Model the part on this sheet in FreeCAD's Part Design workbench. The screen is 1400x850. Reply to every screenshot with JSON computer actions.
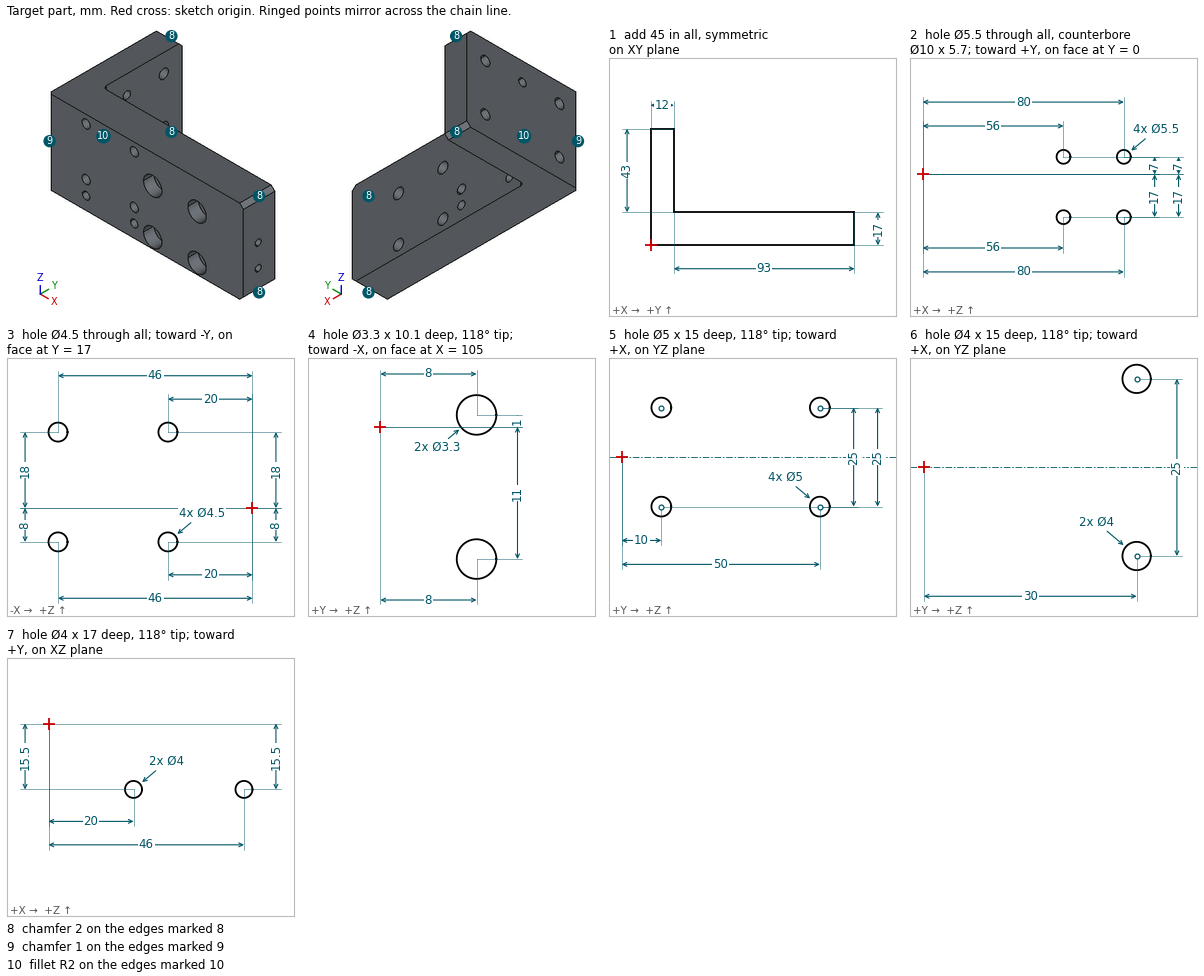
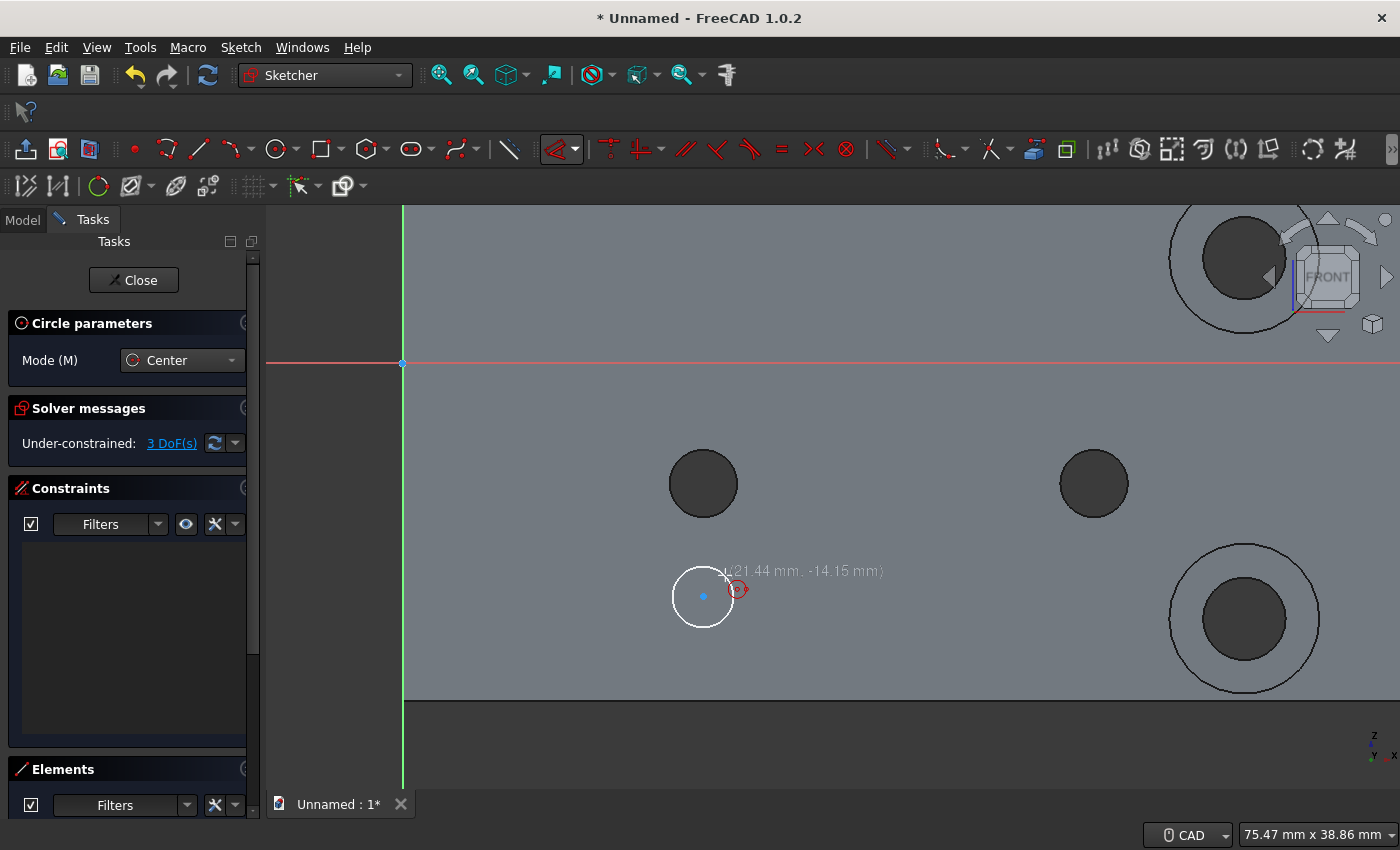
{"action": "left_click", "coordinate": [1094, 596]}
{"action": "left_click", "coordinate": [1115, 575]}
{"action": "key", "text": "Escape"}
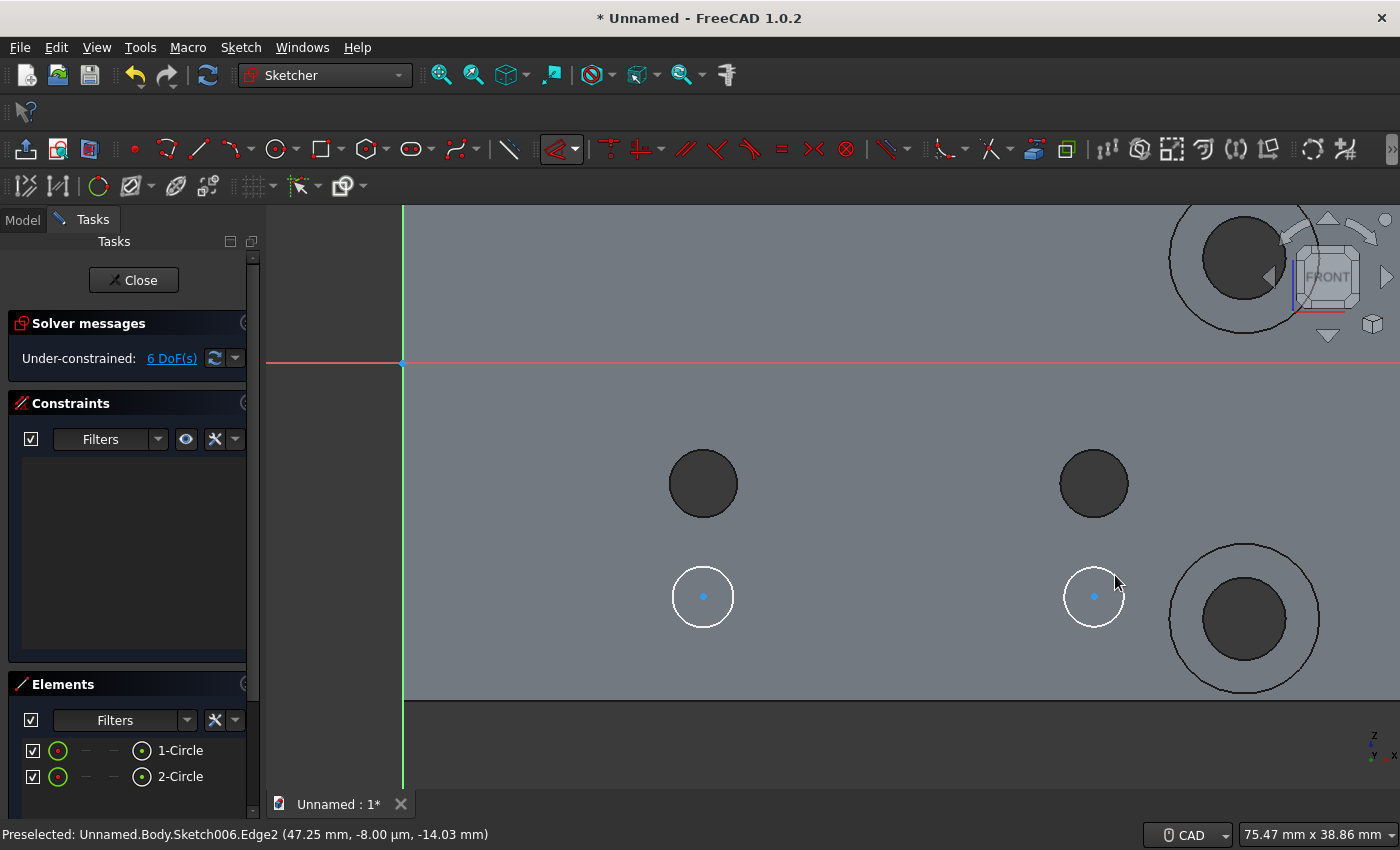
{"action": "left_click", "coordinate": [724, 575]}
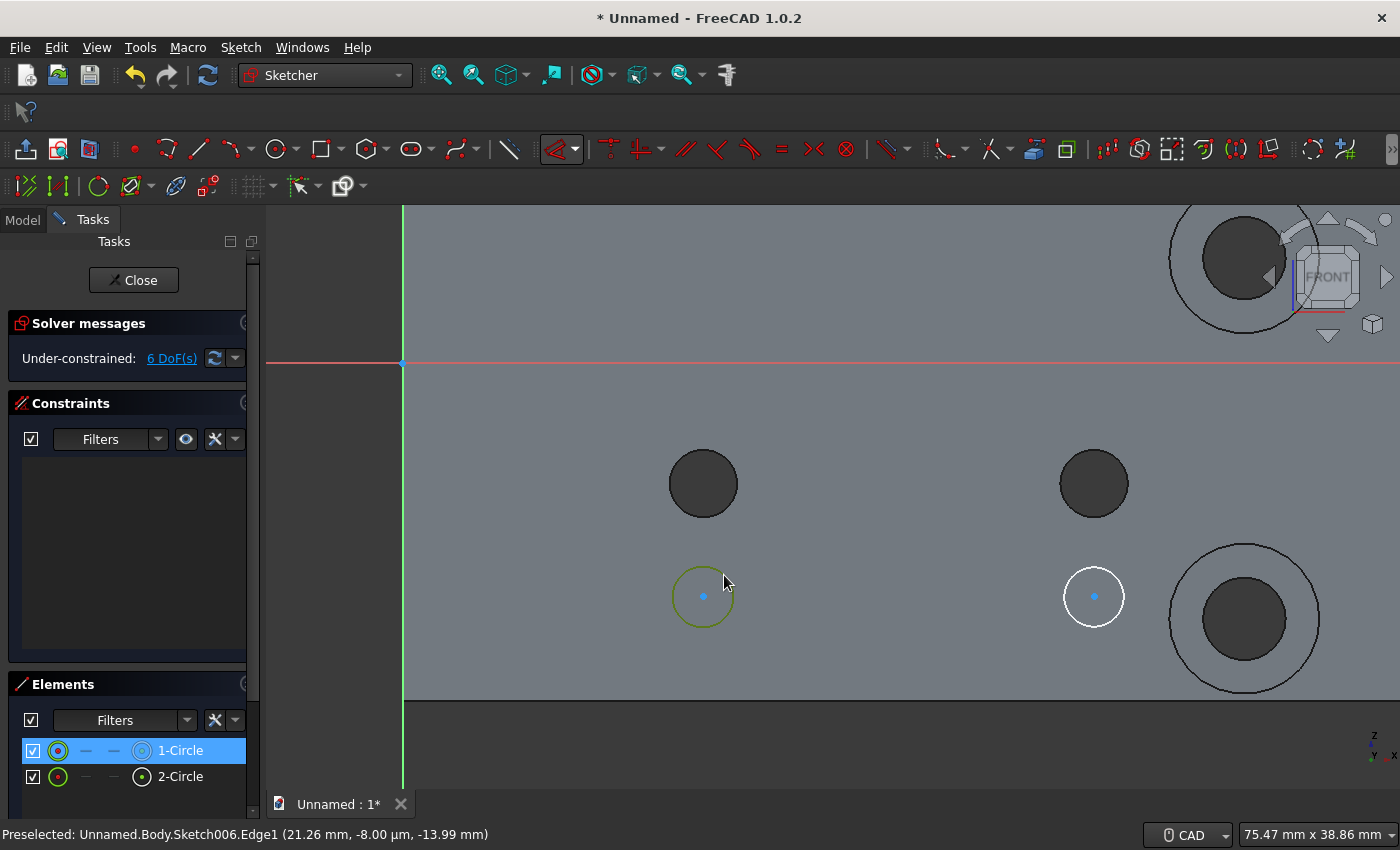
{"action": "left_click", "coordinate": [1115, 576]}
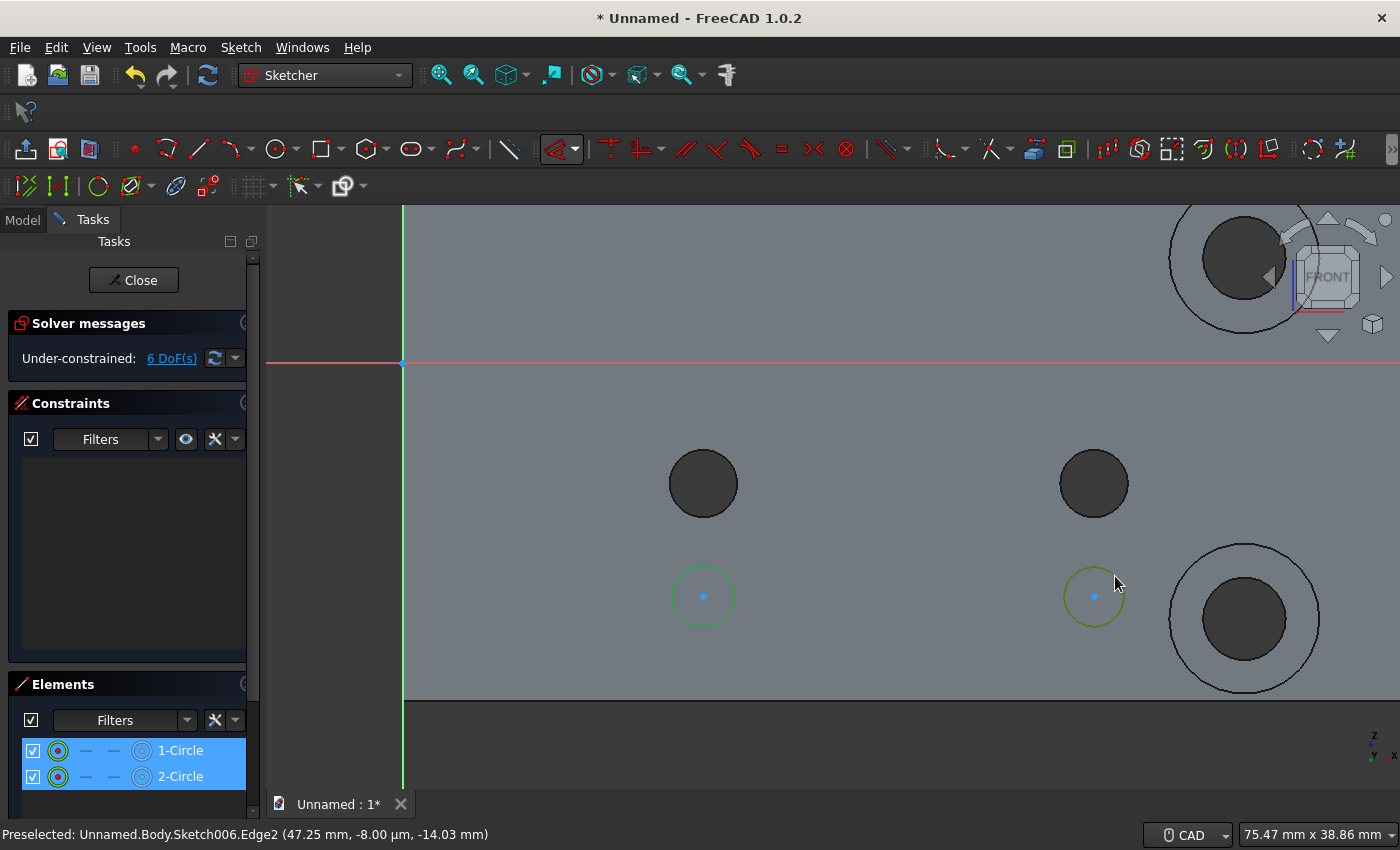
{"action": "key", "text": "e"}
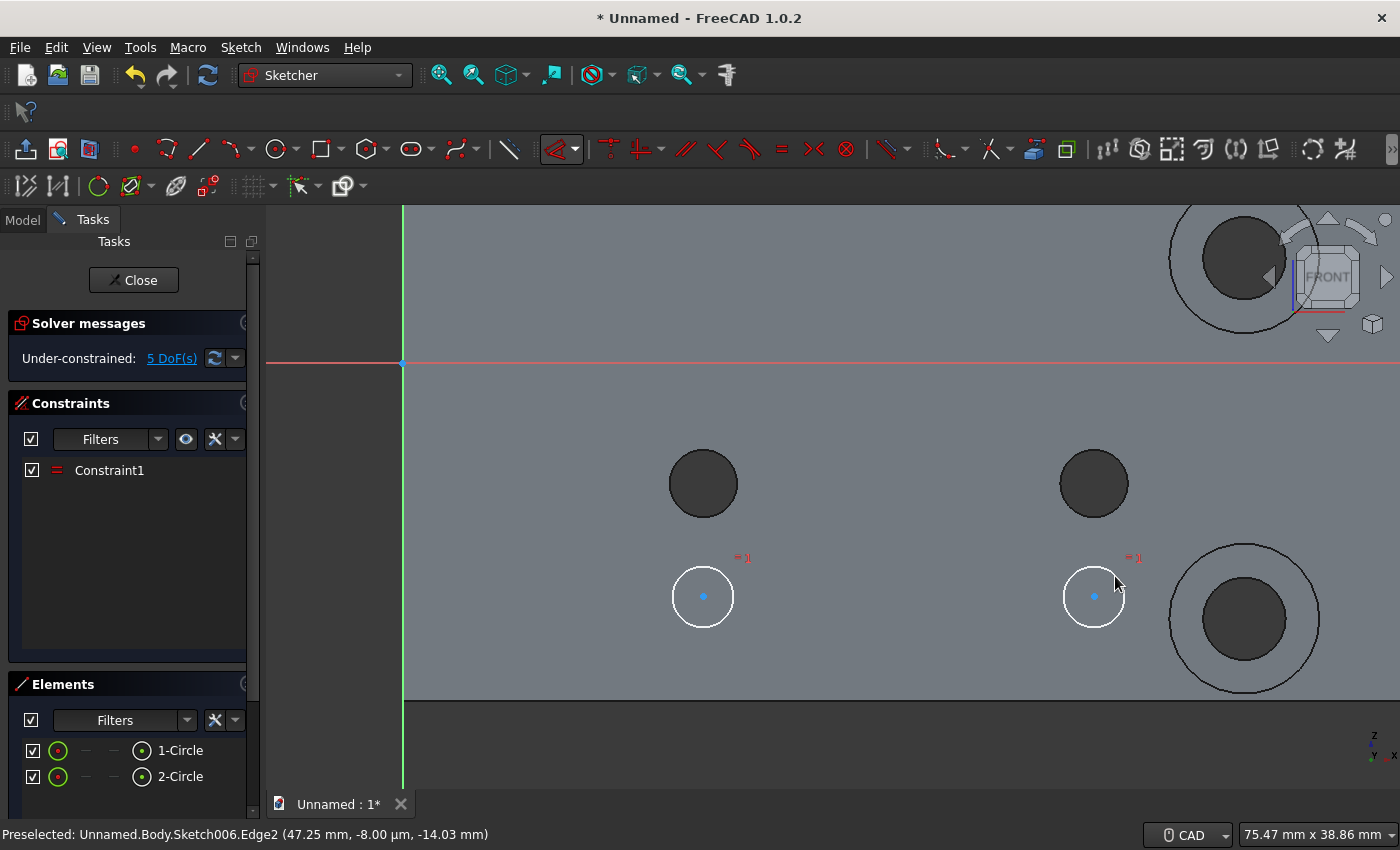
{"action": "left_click", "coordinate": [724, 575]}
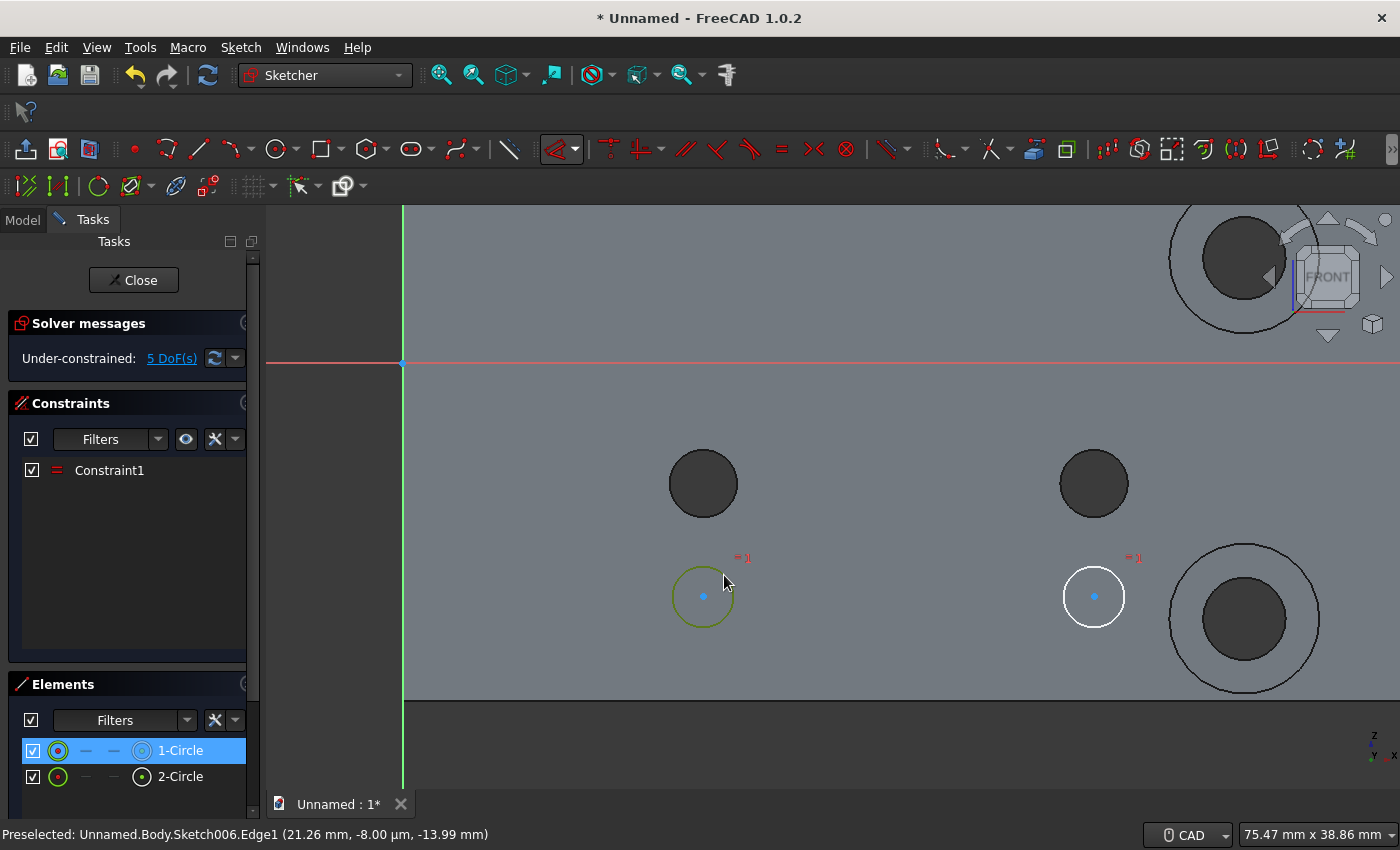
{"action": "key", "text": "k o"}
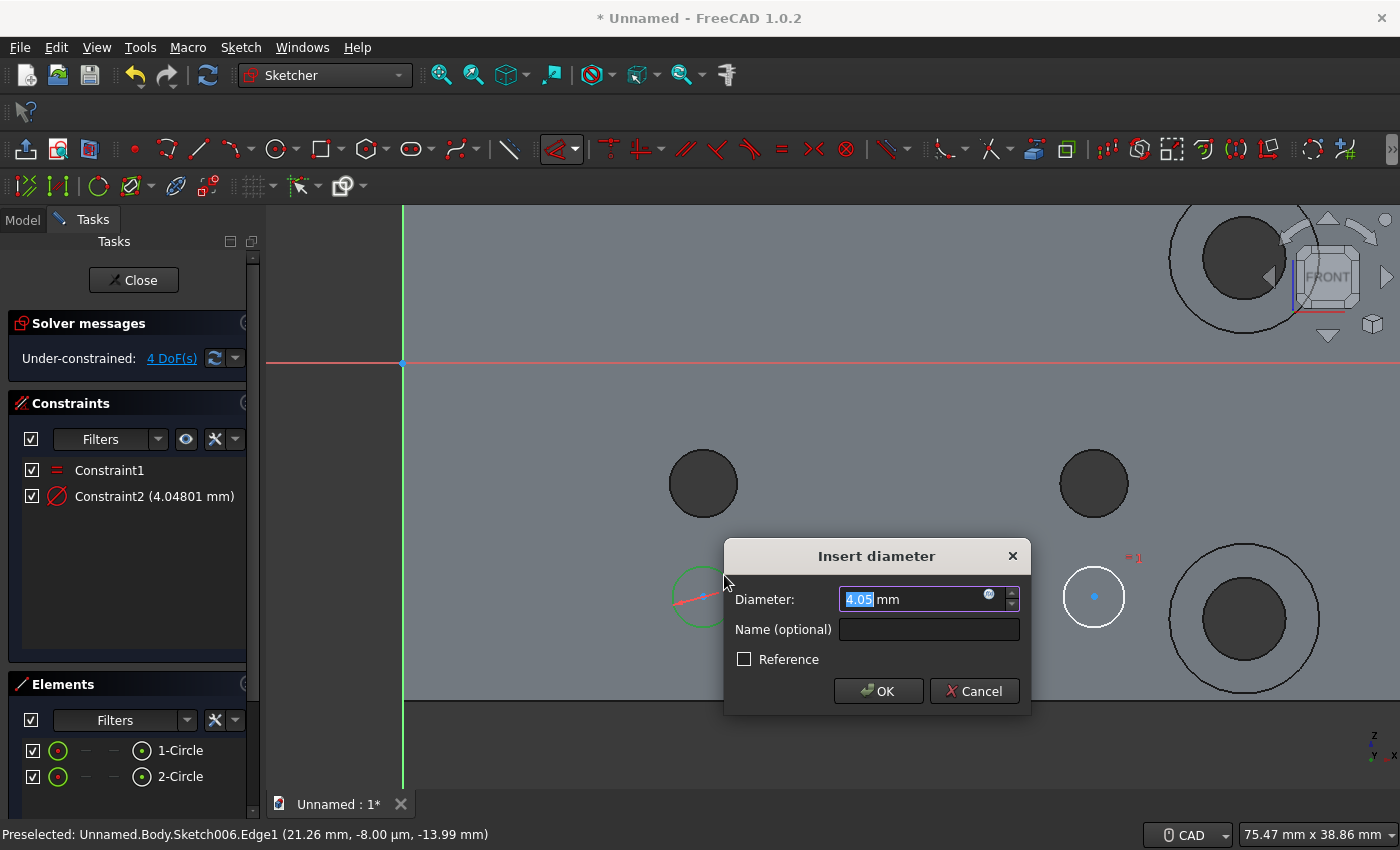
{"action": "type", "text": "4"}
{"action": "key", "text": "Return"}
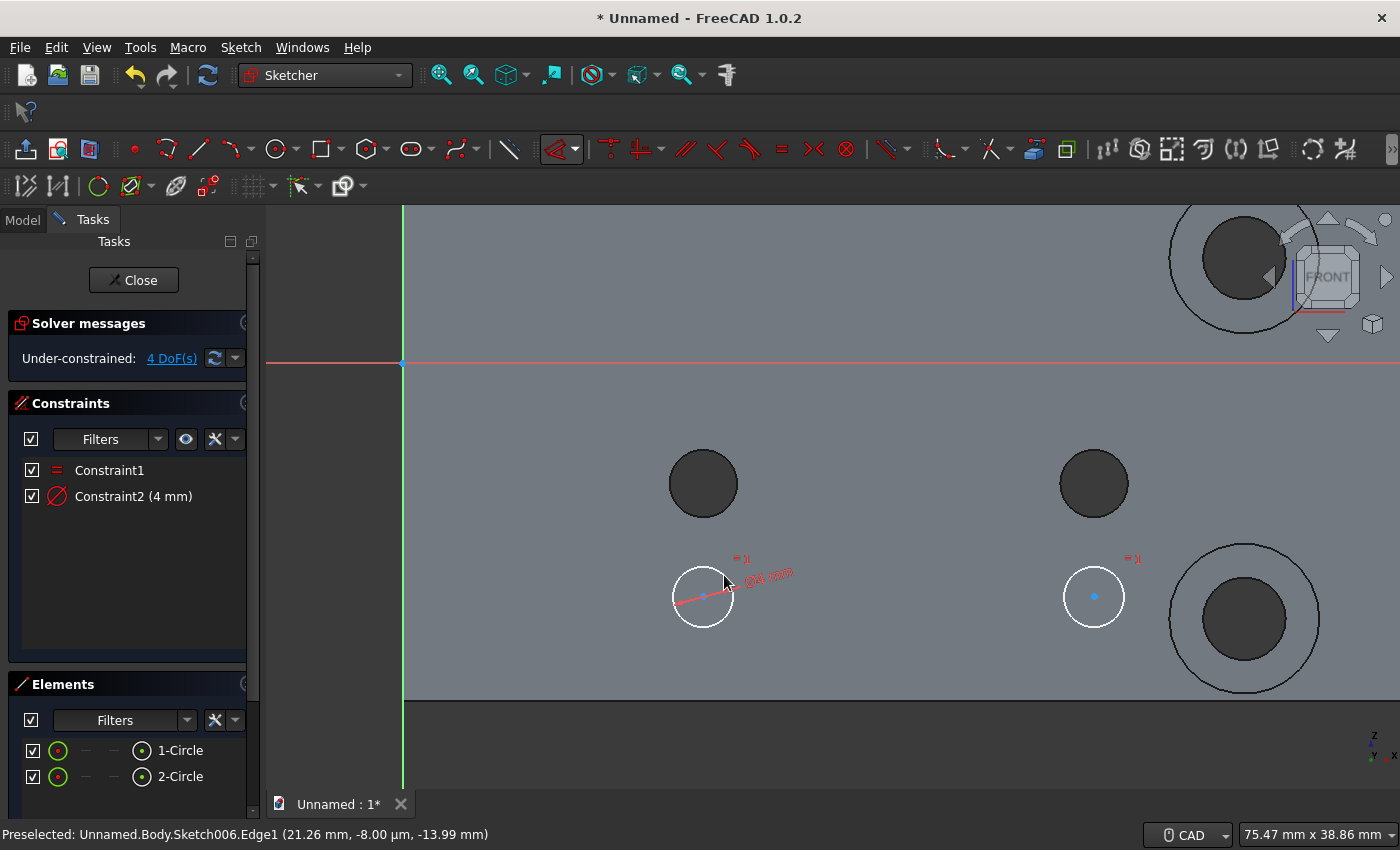
{"action": "left_click", "coordinate": [703, 597]}